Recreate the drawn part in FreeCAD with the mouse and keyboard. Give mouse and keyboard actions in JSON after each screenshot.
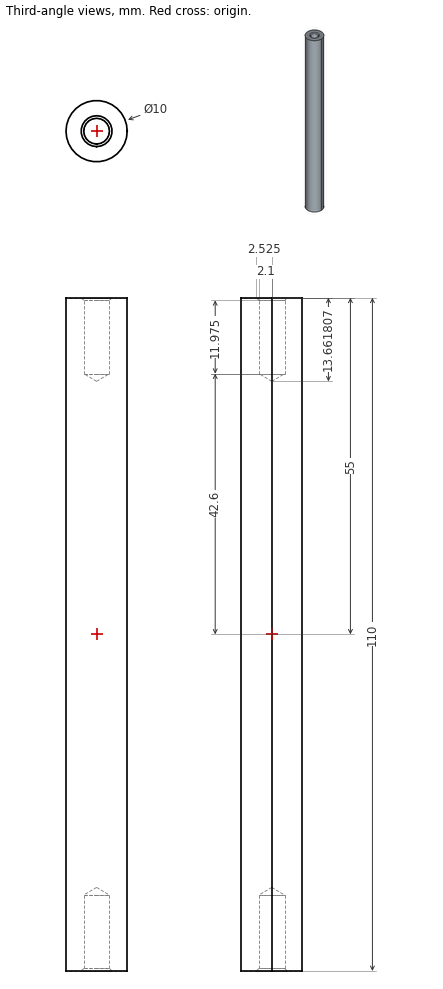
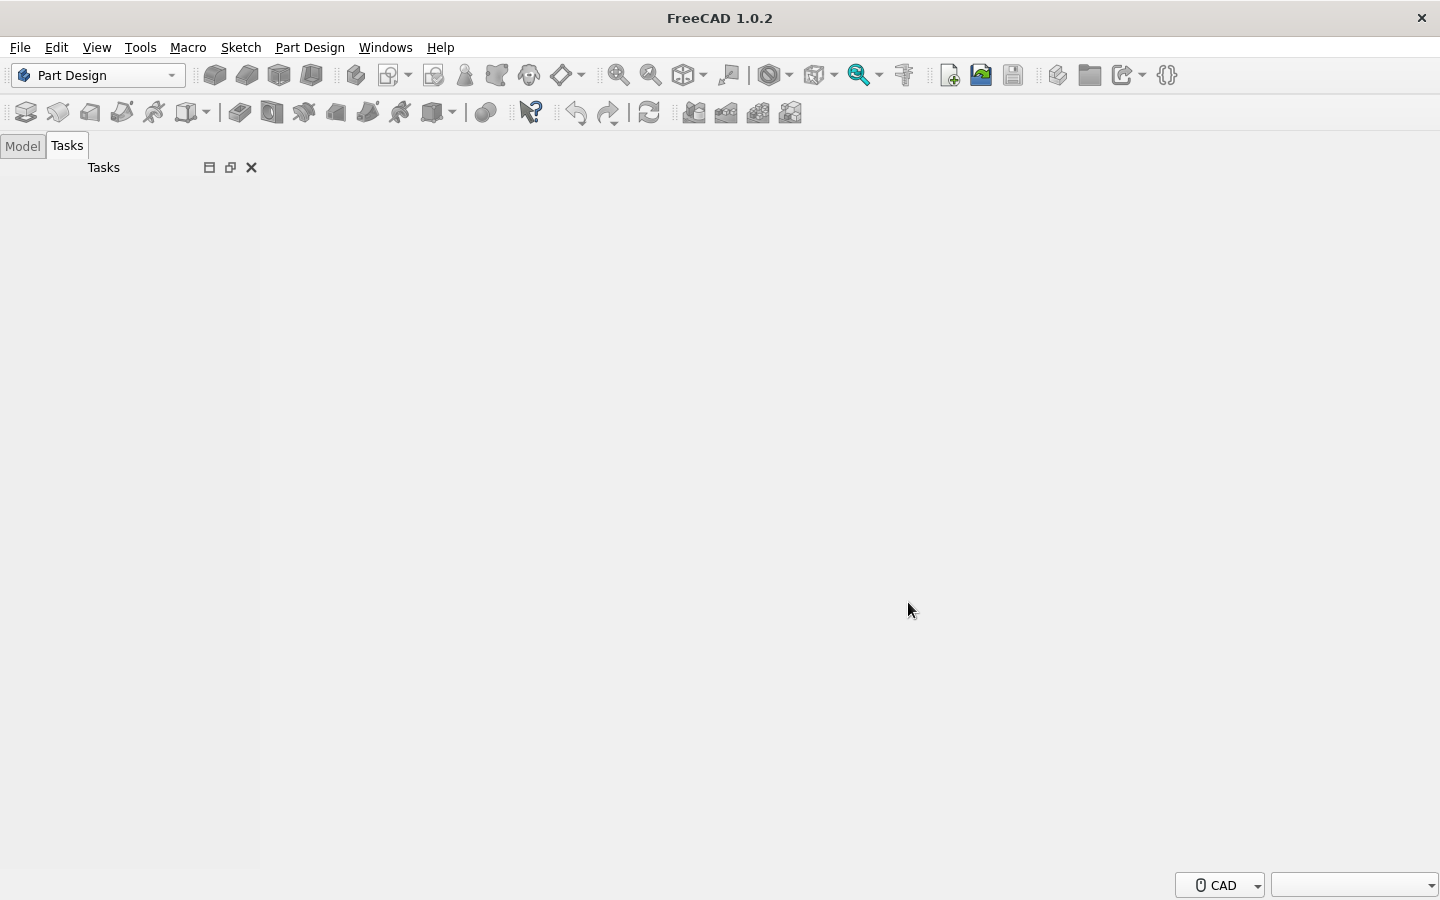
{"action": "left_click", "coordinate": [950, 76]}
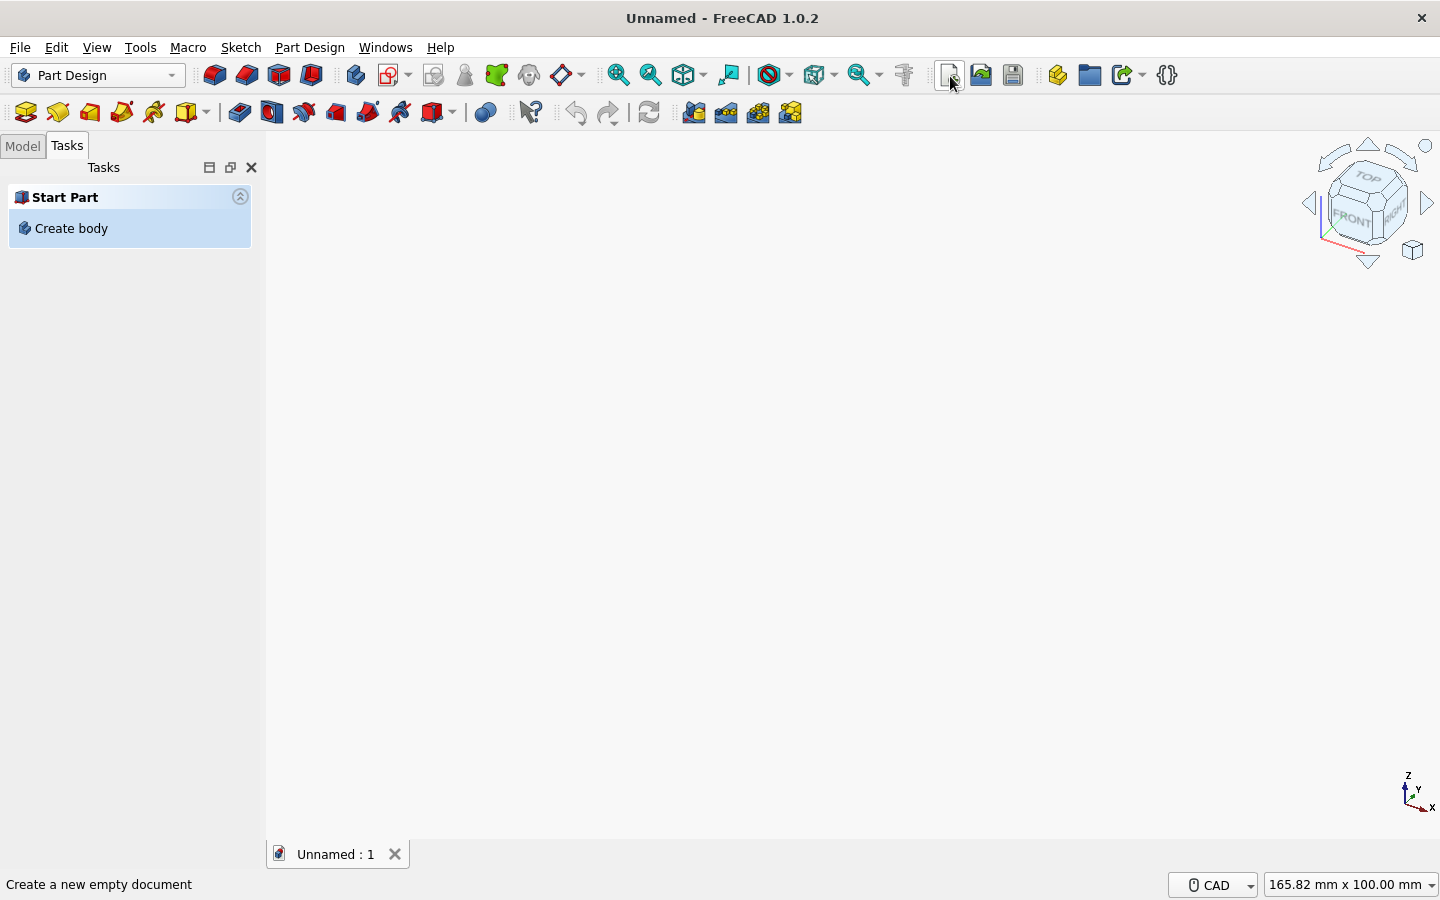
{"action": "left_click", "coordinate": [388, 76]}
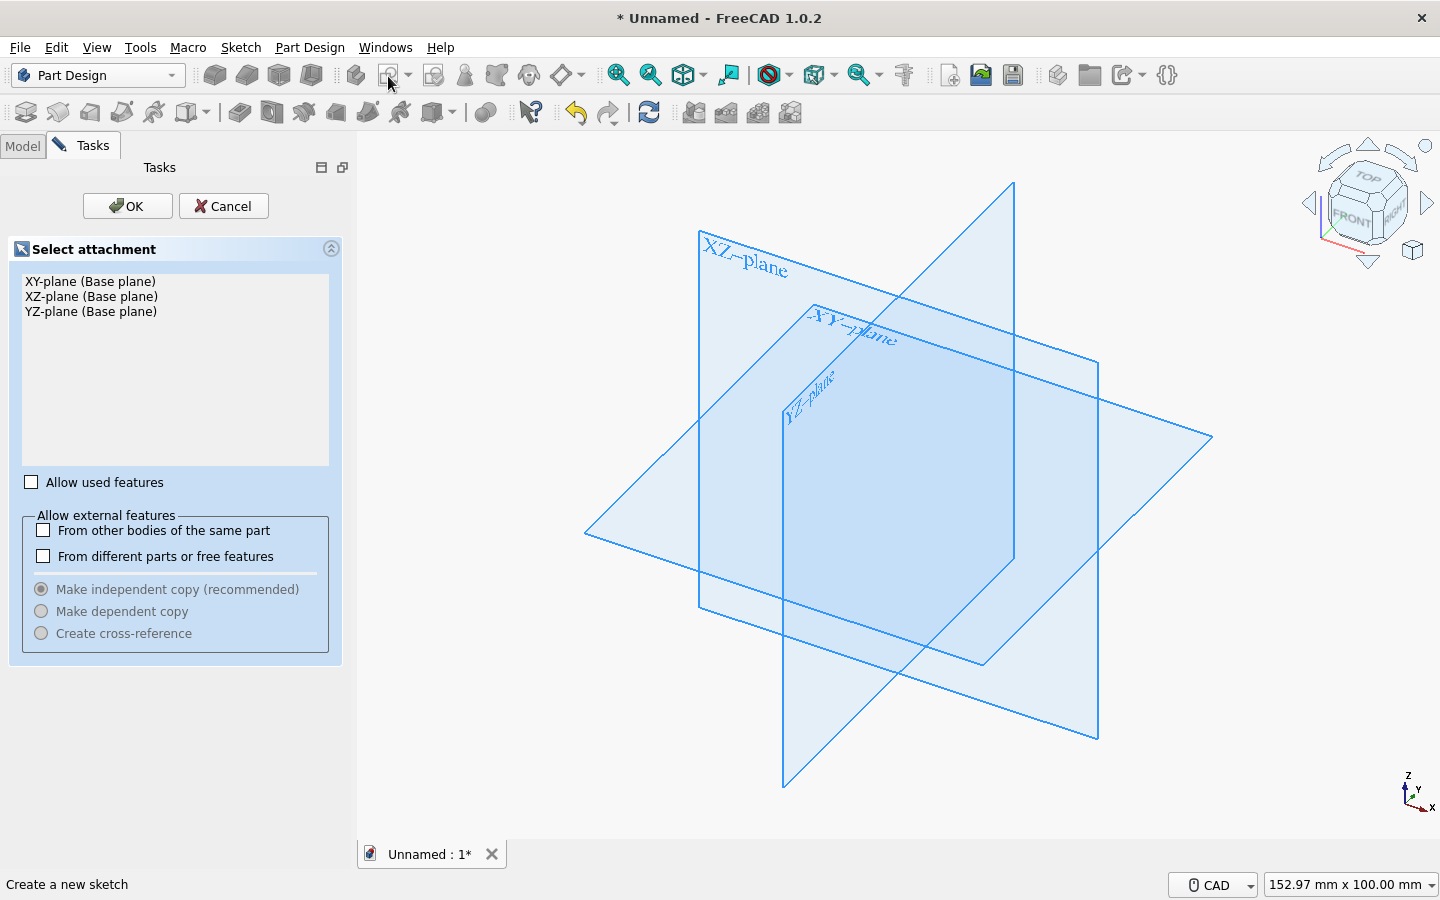
{"action": "left_click", "coordinate": [82, 282]}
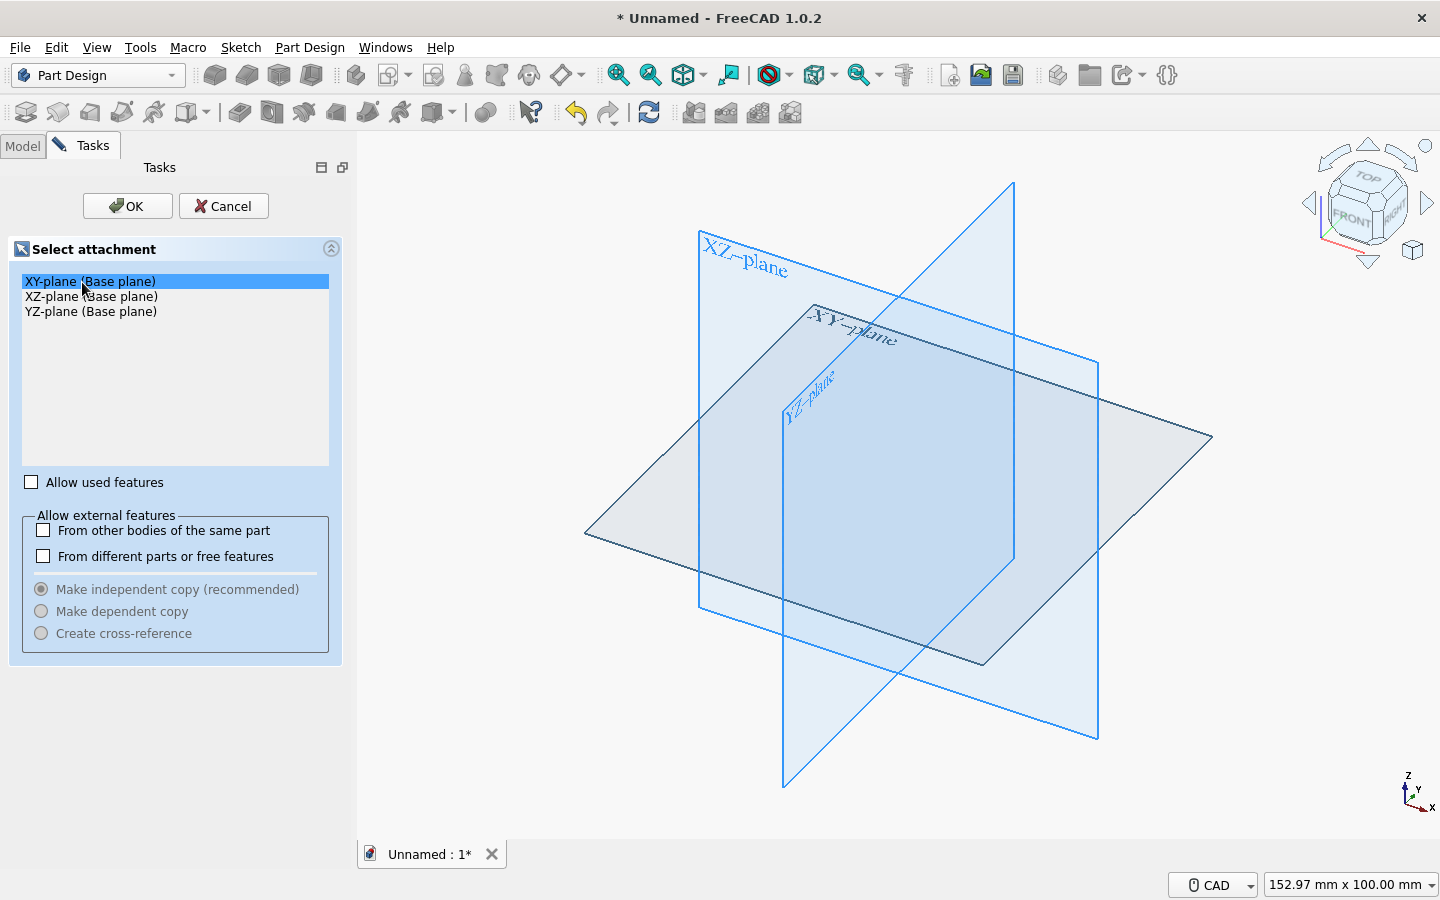
{"action": "left_click", "coordinate": [128, 206]}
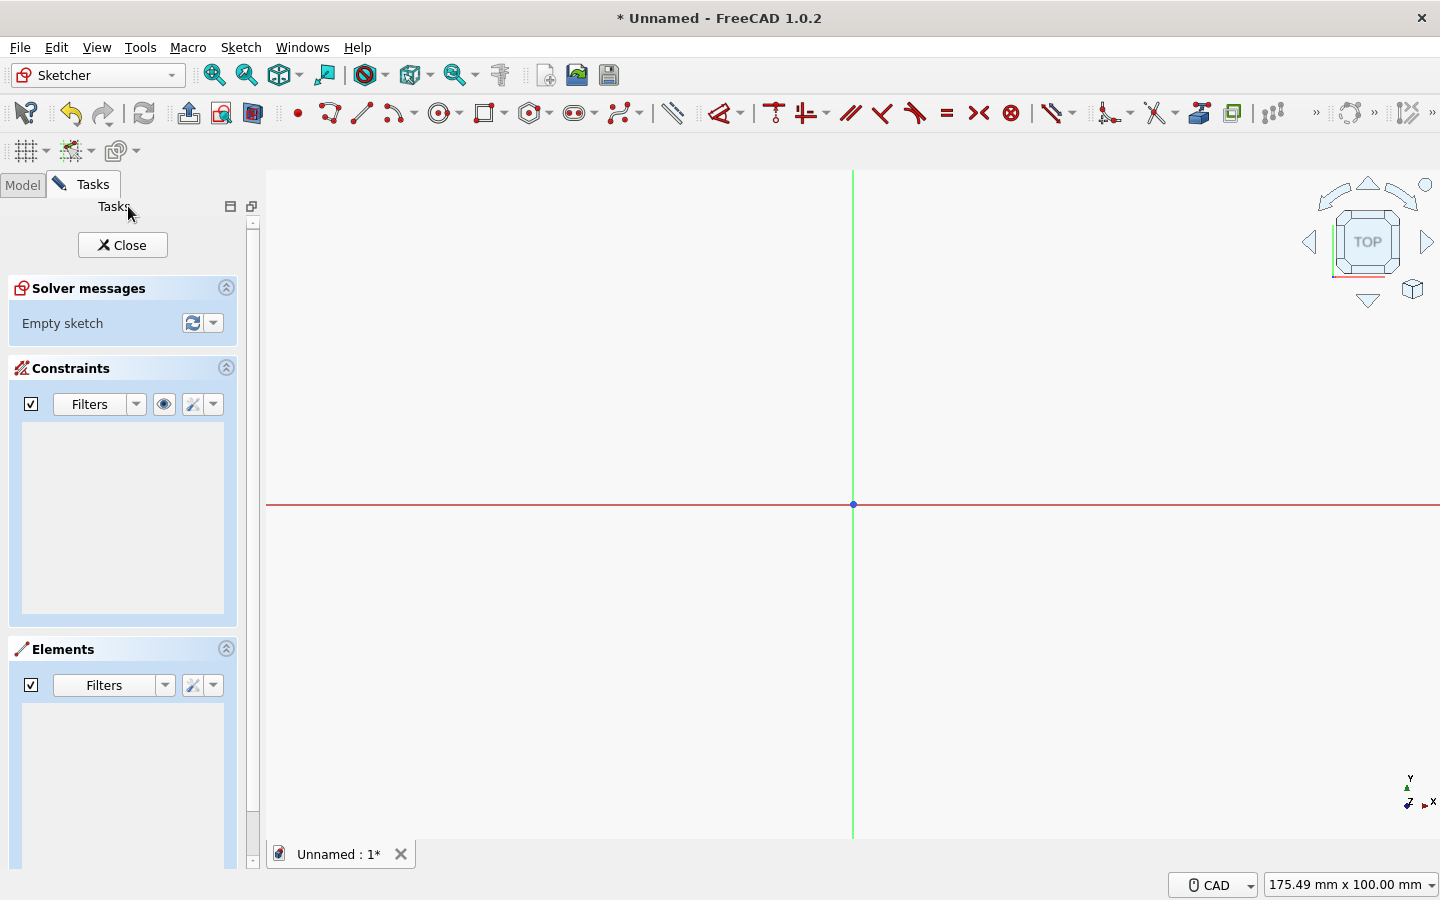
{"action": "scroll", "coordinate": [867, 505], "scroll_direction": "up", "scroll_amount": 9}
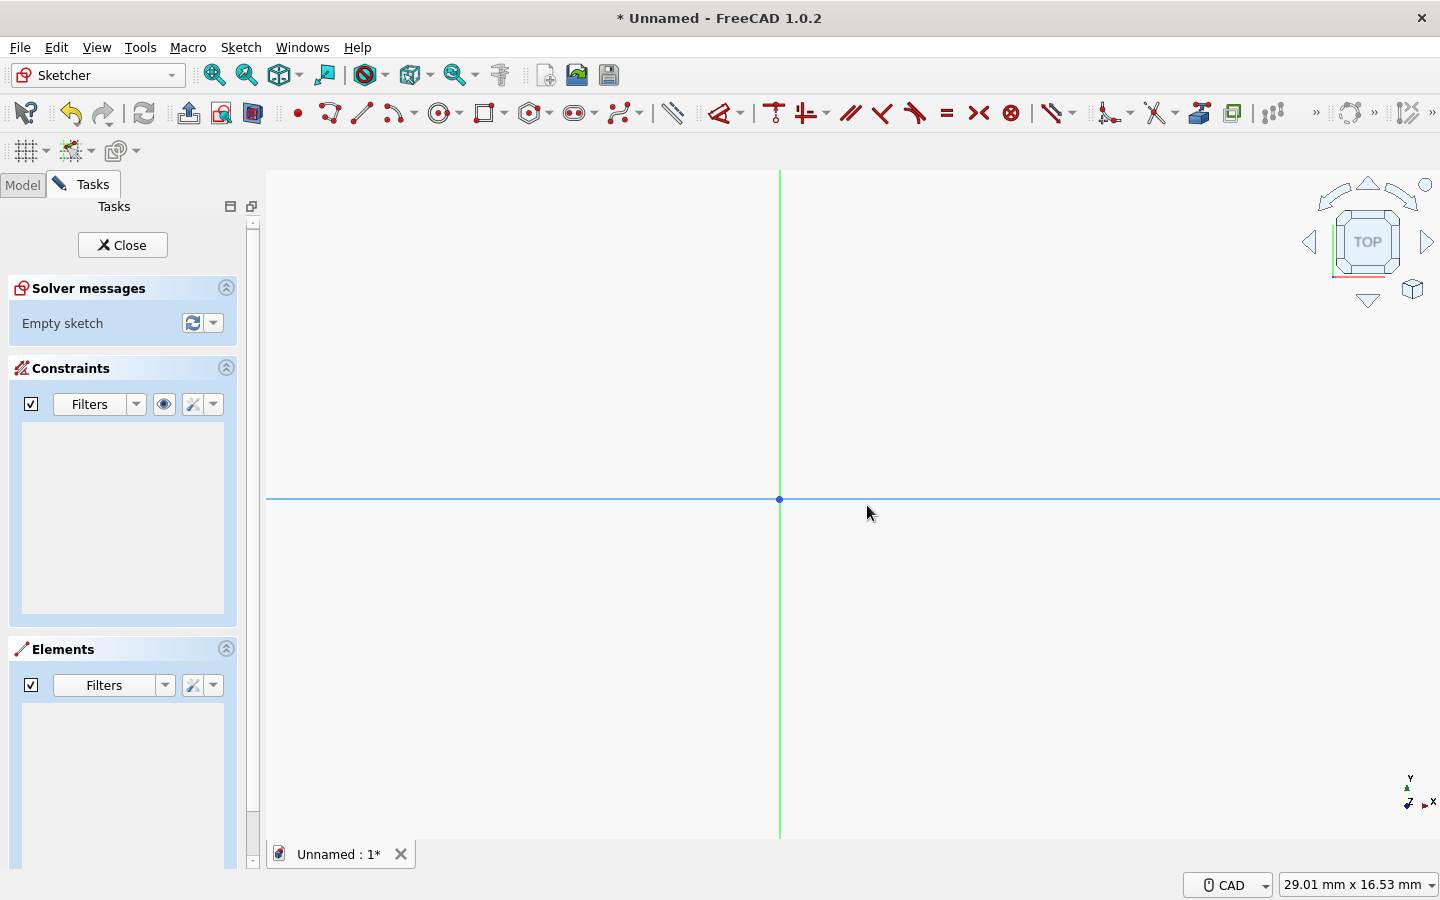
{"action": "left_click", "coordinate": [440, 114]}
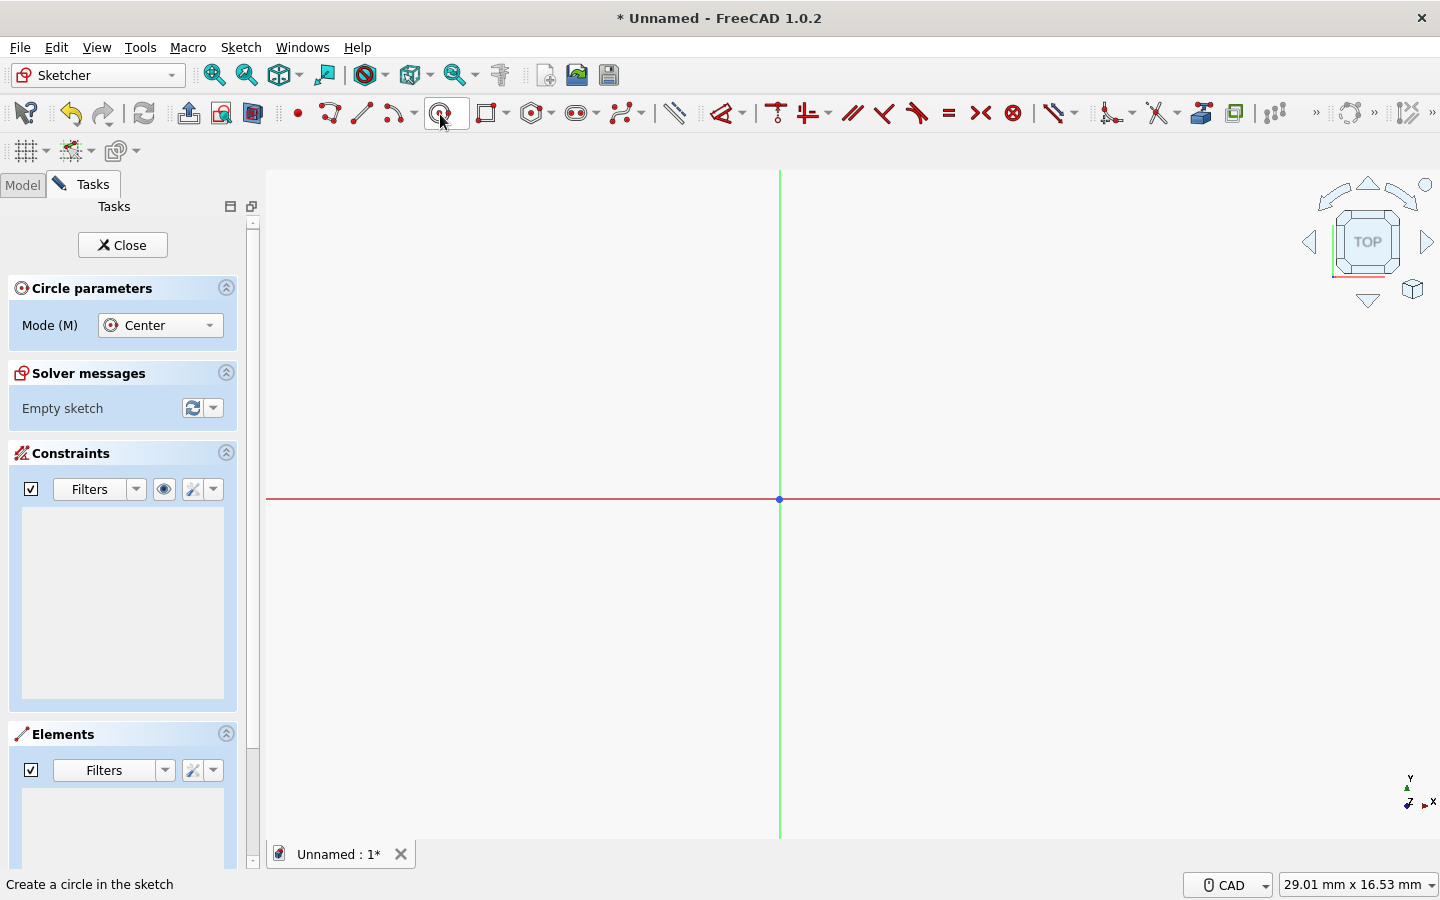
{"action": "left_click", "coordinate": [780, 499]}
{"action": "mouse_move", "coordinate": [923, 356]}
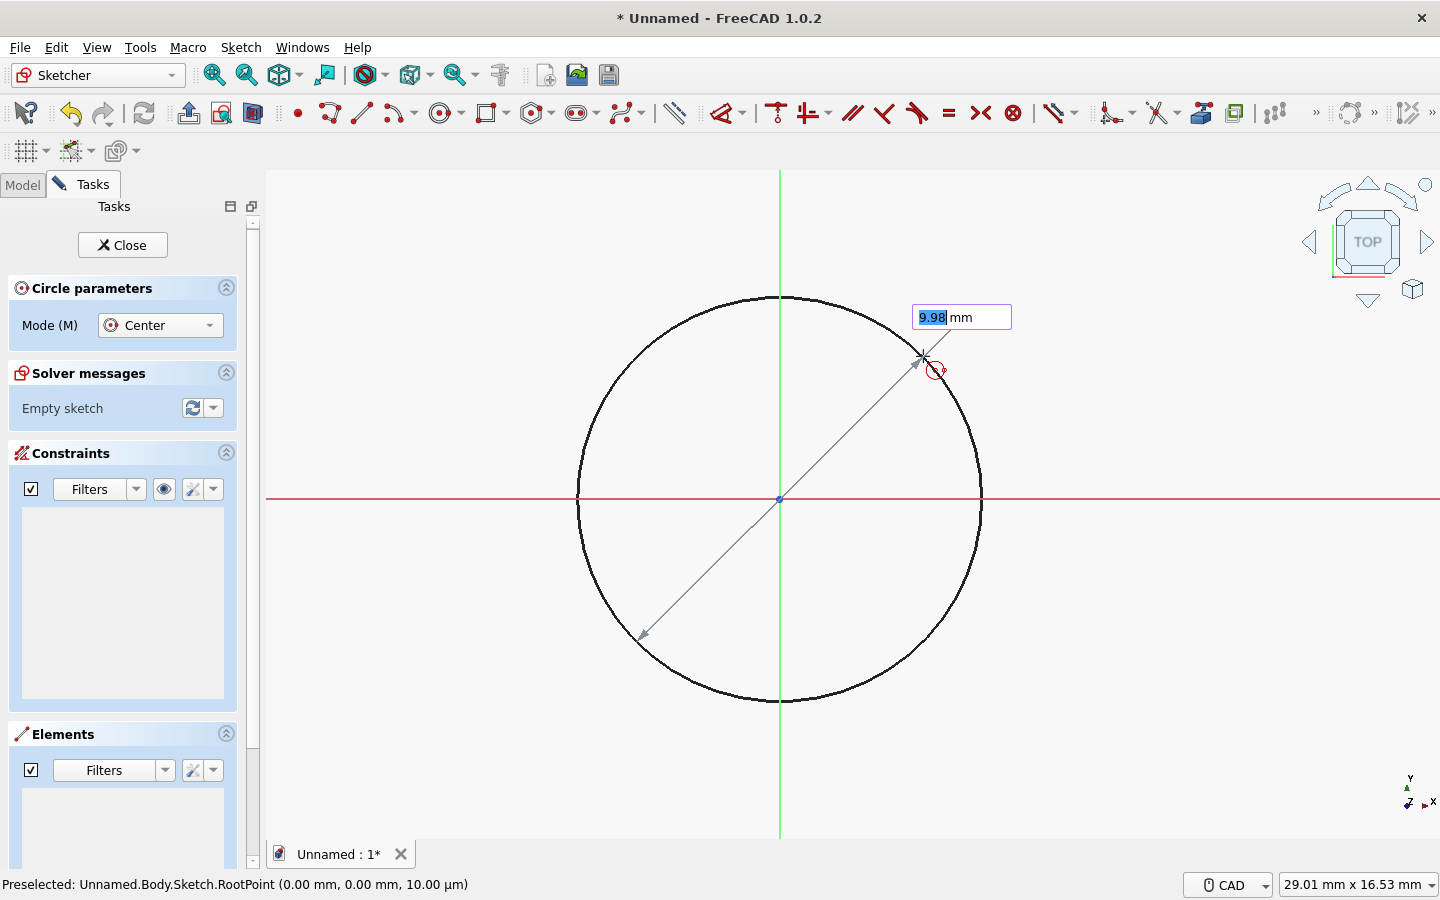
{"action": "type", "text": "10"}
{"action": "key", "text": "Return"}
{"action": "key", "text": "Escape"}